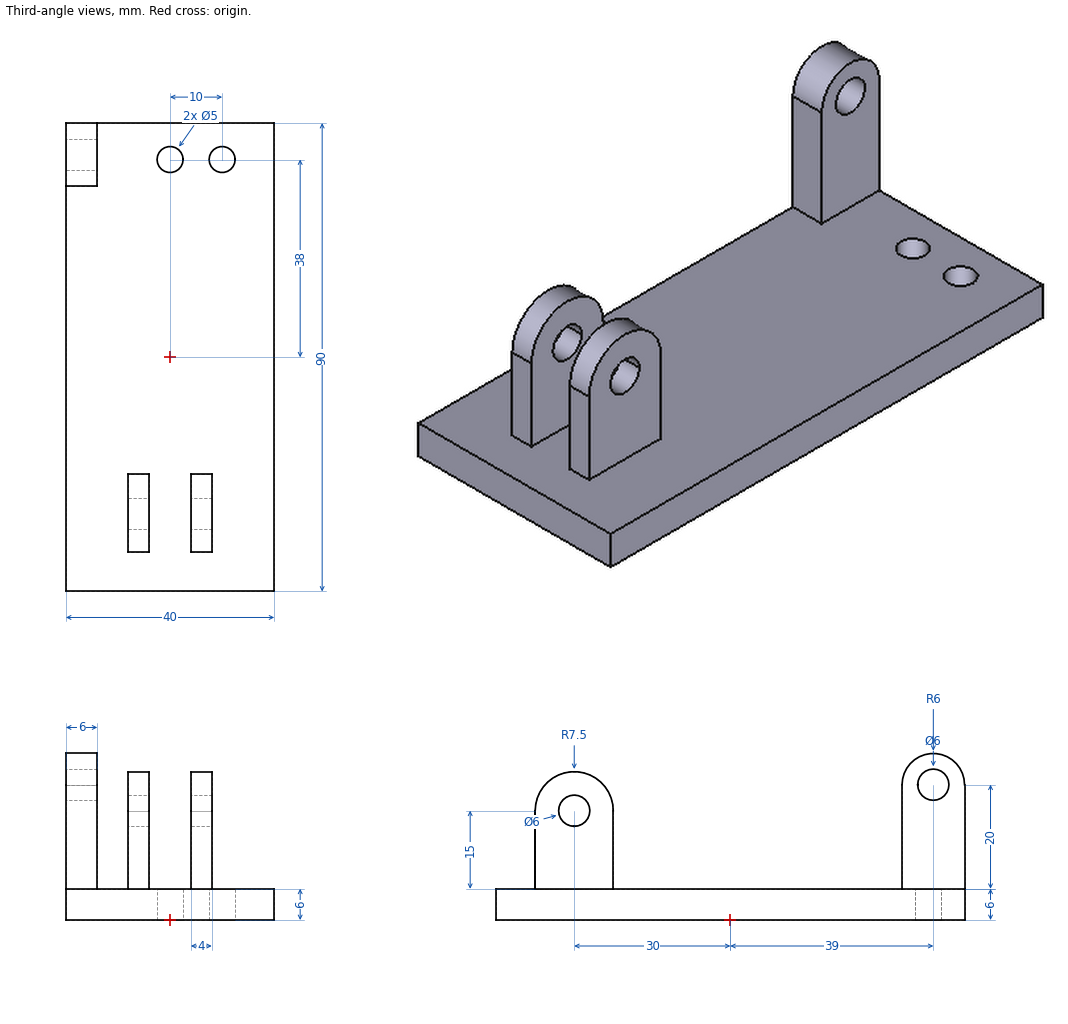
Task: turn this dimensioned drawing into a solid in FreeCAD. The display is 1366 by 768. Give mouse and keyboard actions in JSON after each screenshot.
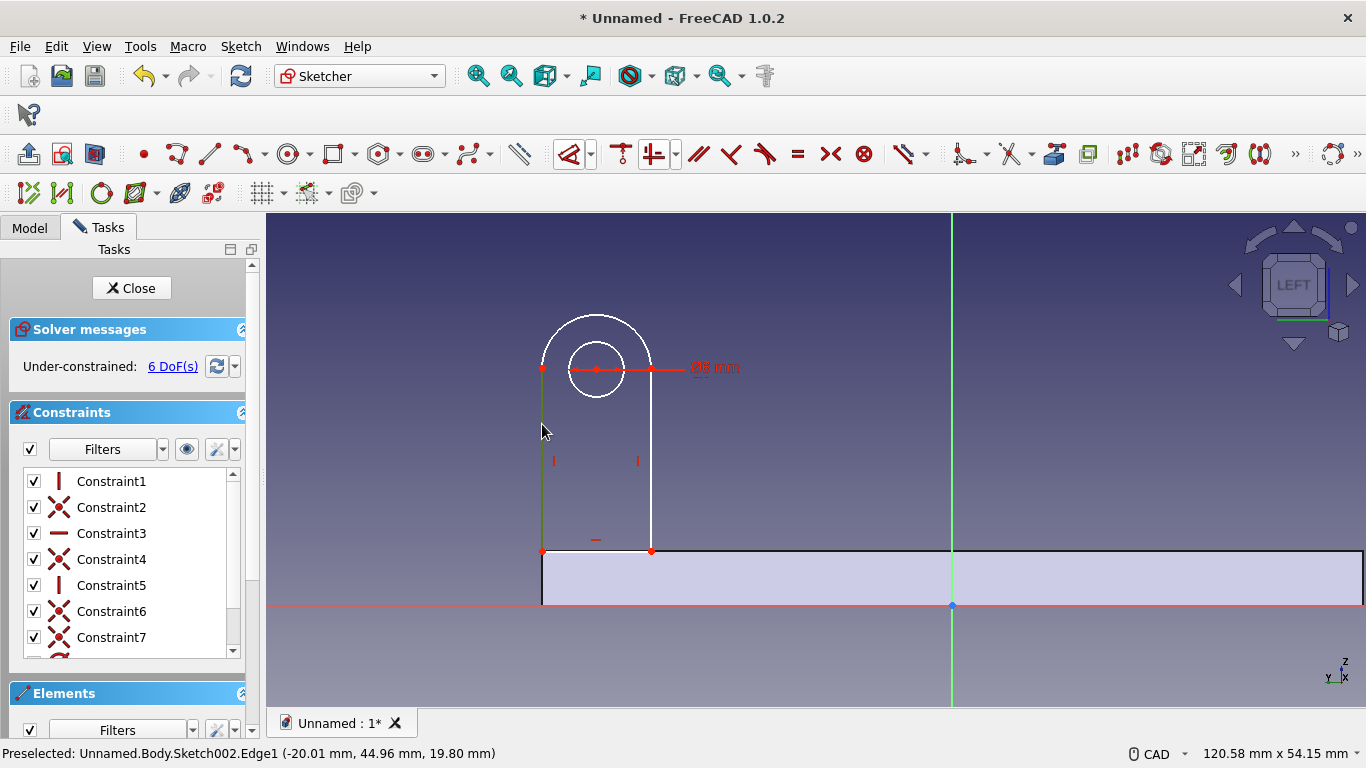
{"action": "left_click", "coordinate": [628, 325]}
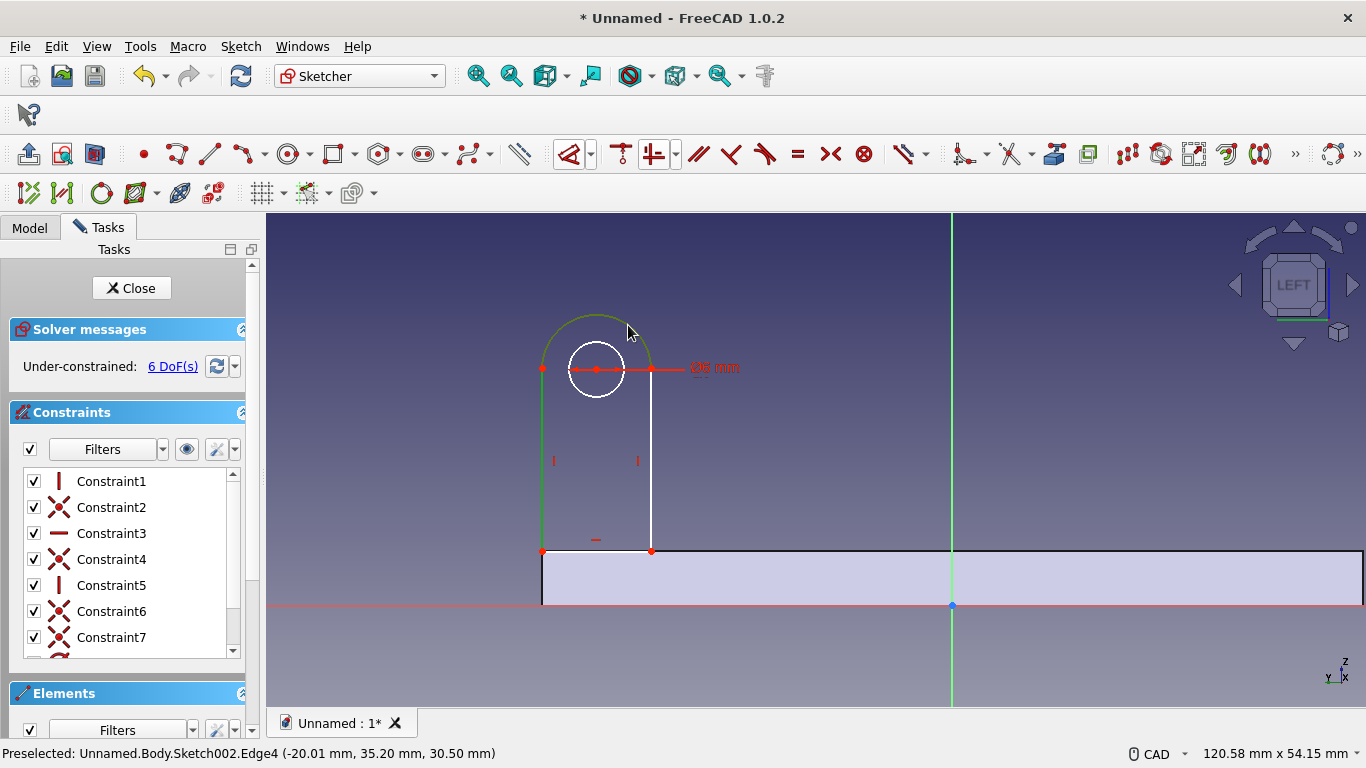
{"action": "key", "text": "t"}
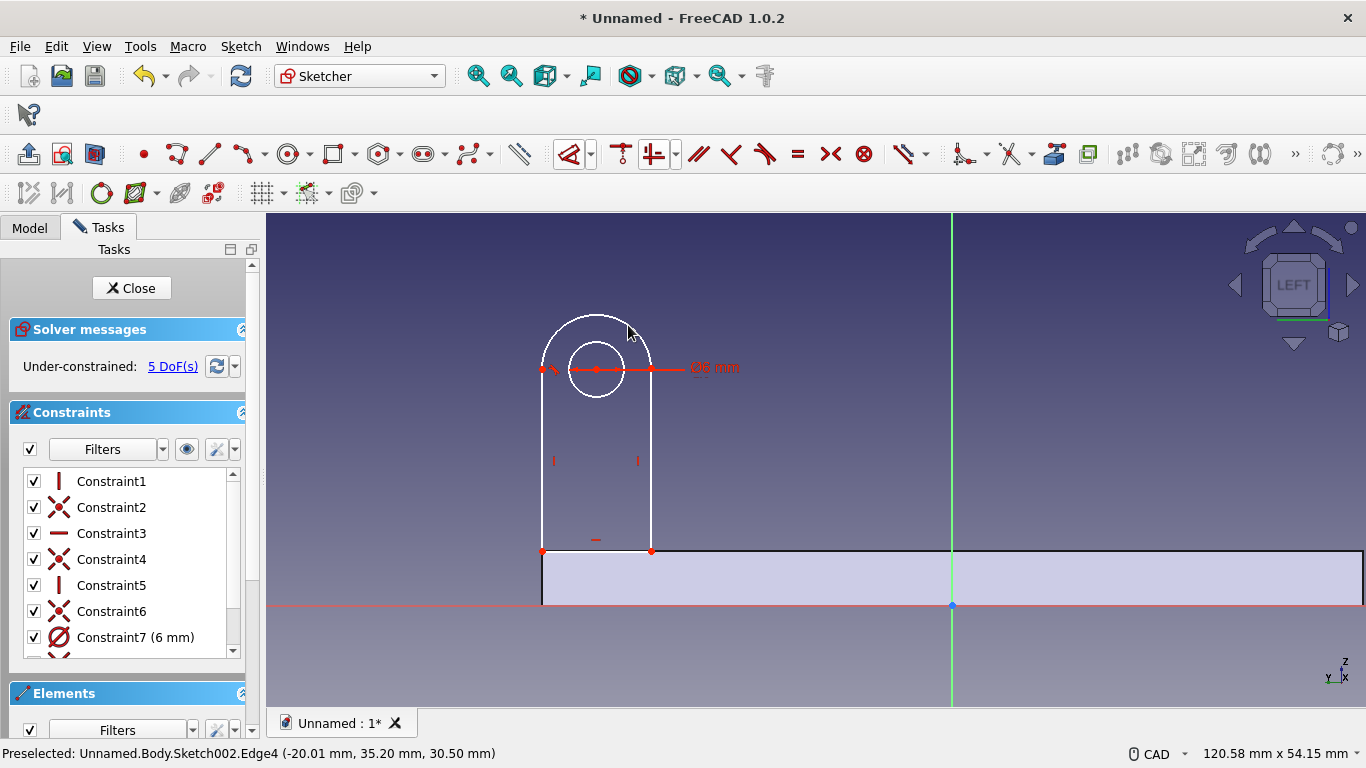
{"action": "left_click", "coordinate": [651, 497]}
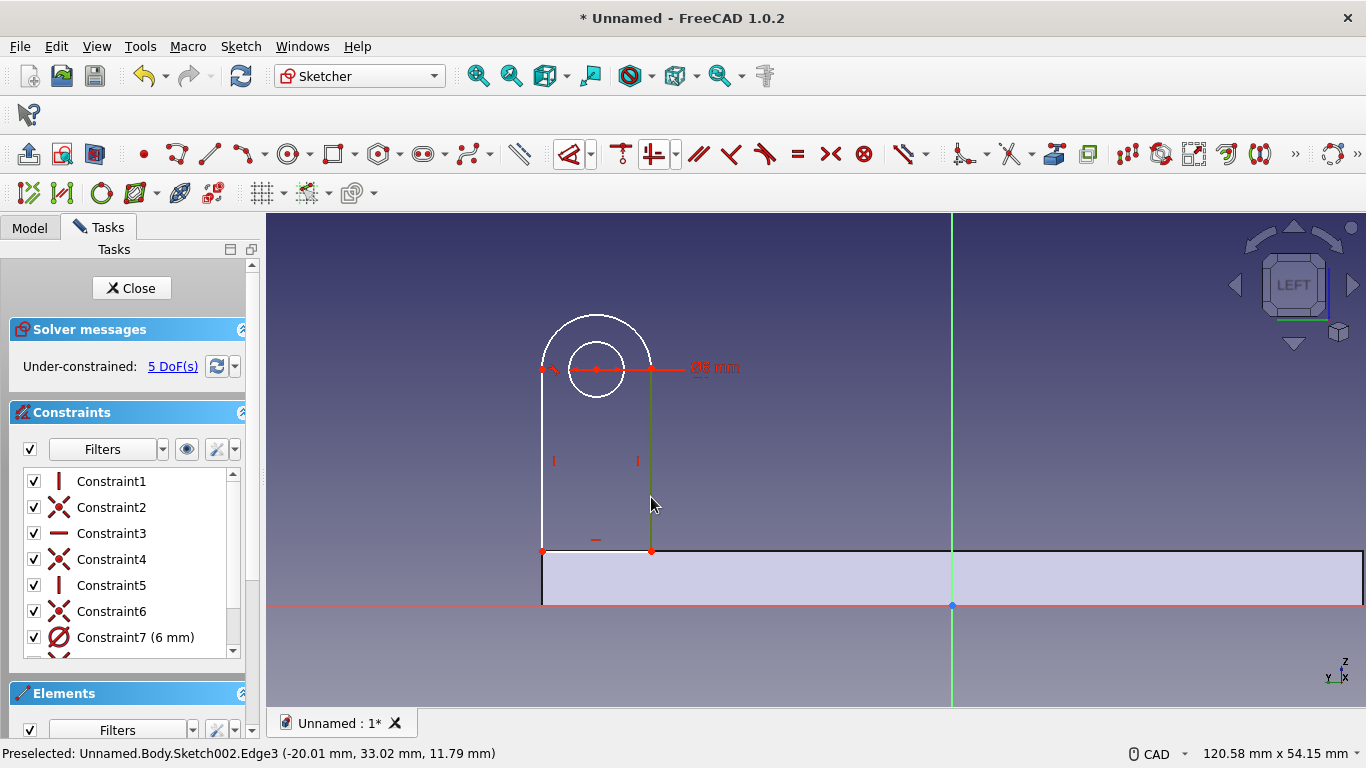
{"action": "left_click", "coordinate": [628, 325]}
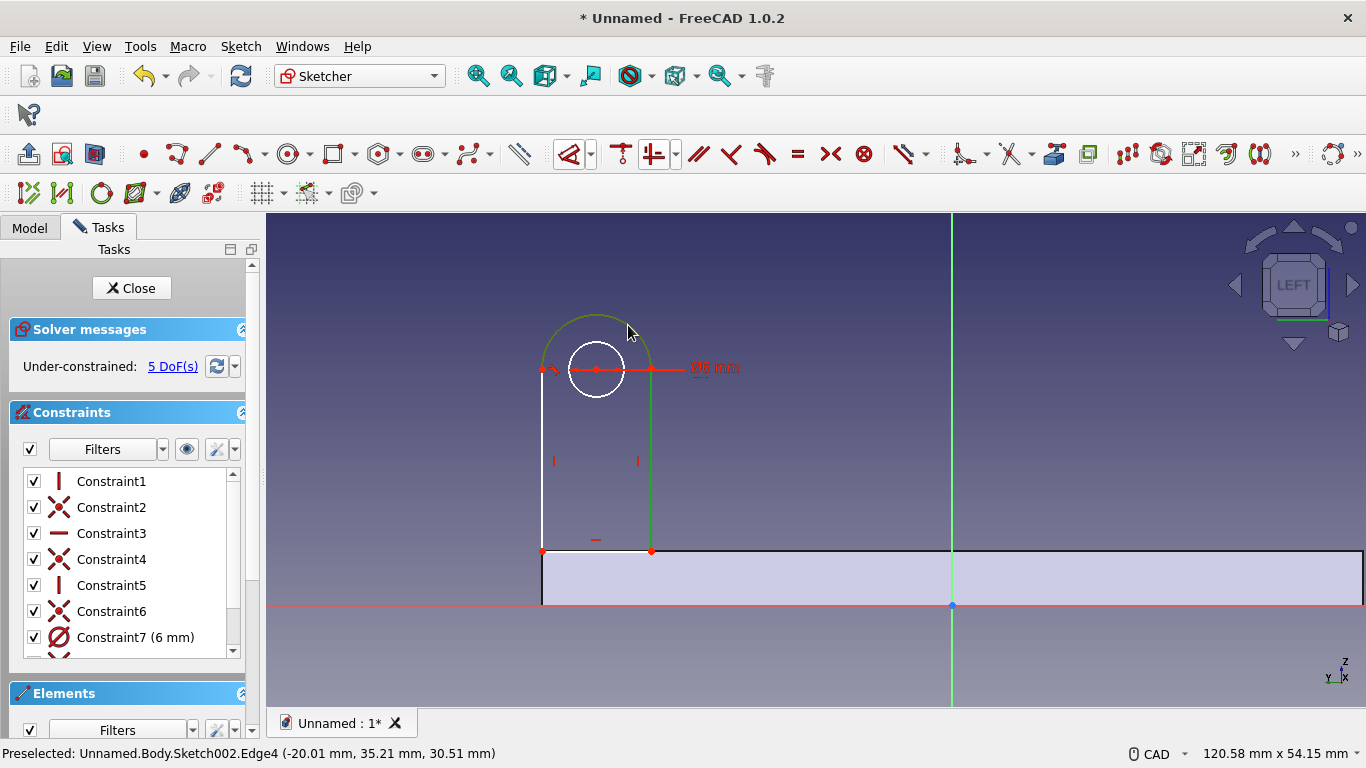
{"action": "key", "text": "t"}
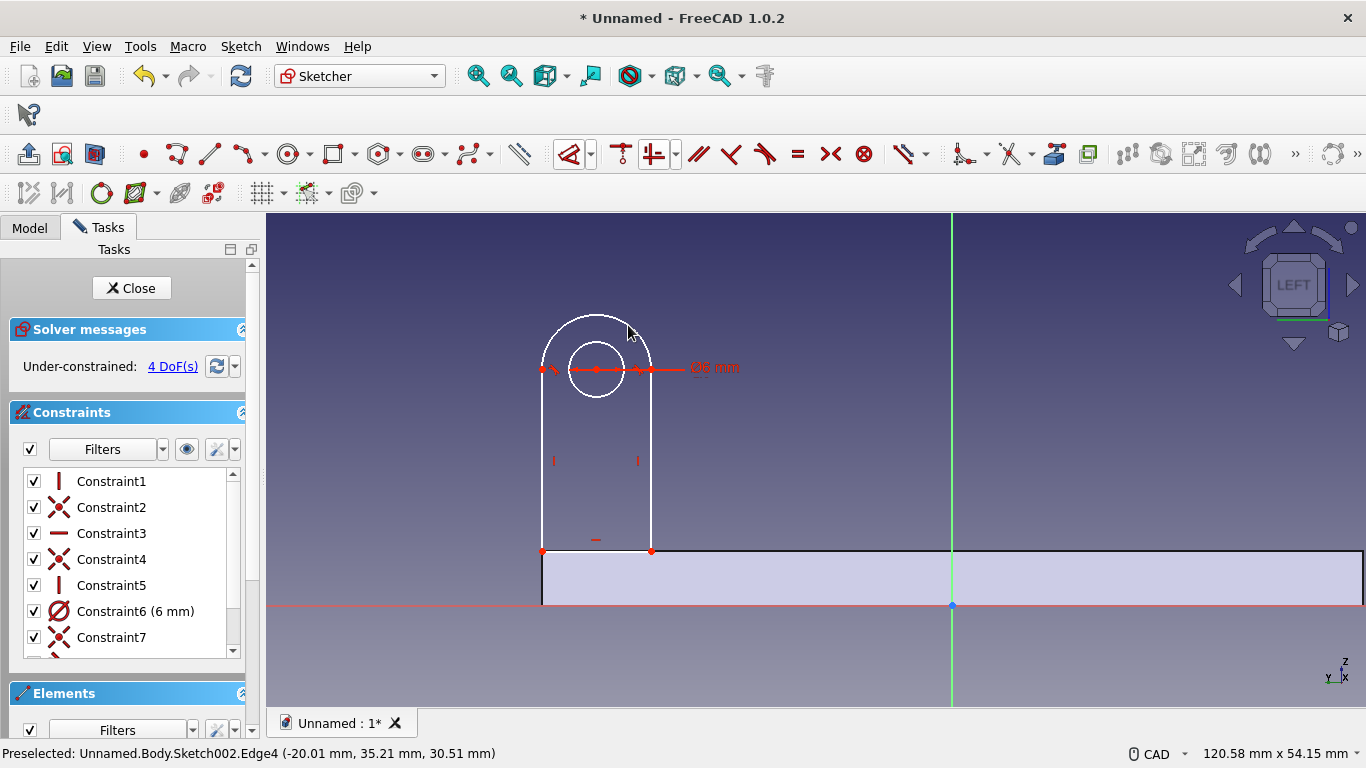
{"action": "key", "text": "d"}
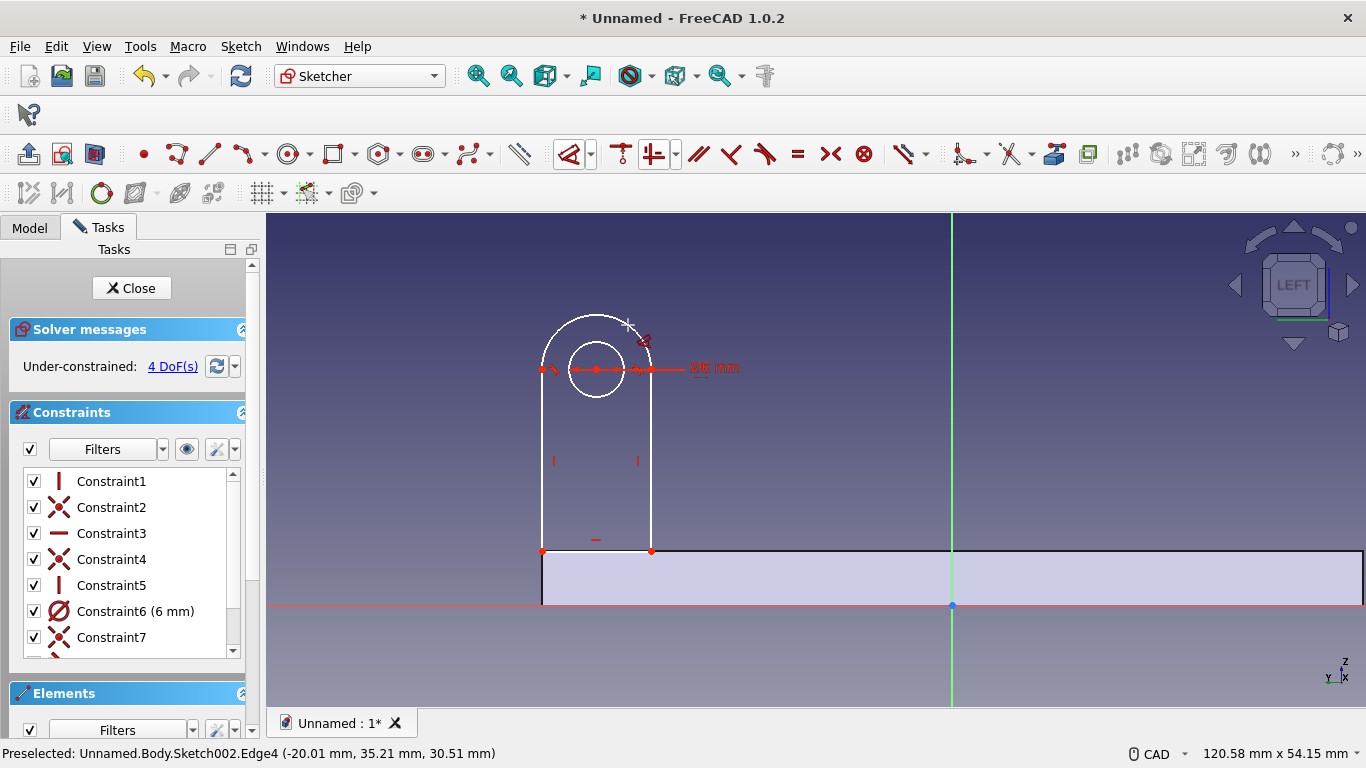
{"action": "left_click", "coordinate": [629, 325]}
{"action": "left_click", "coordinate": [648, 299]}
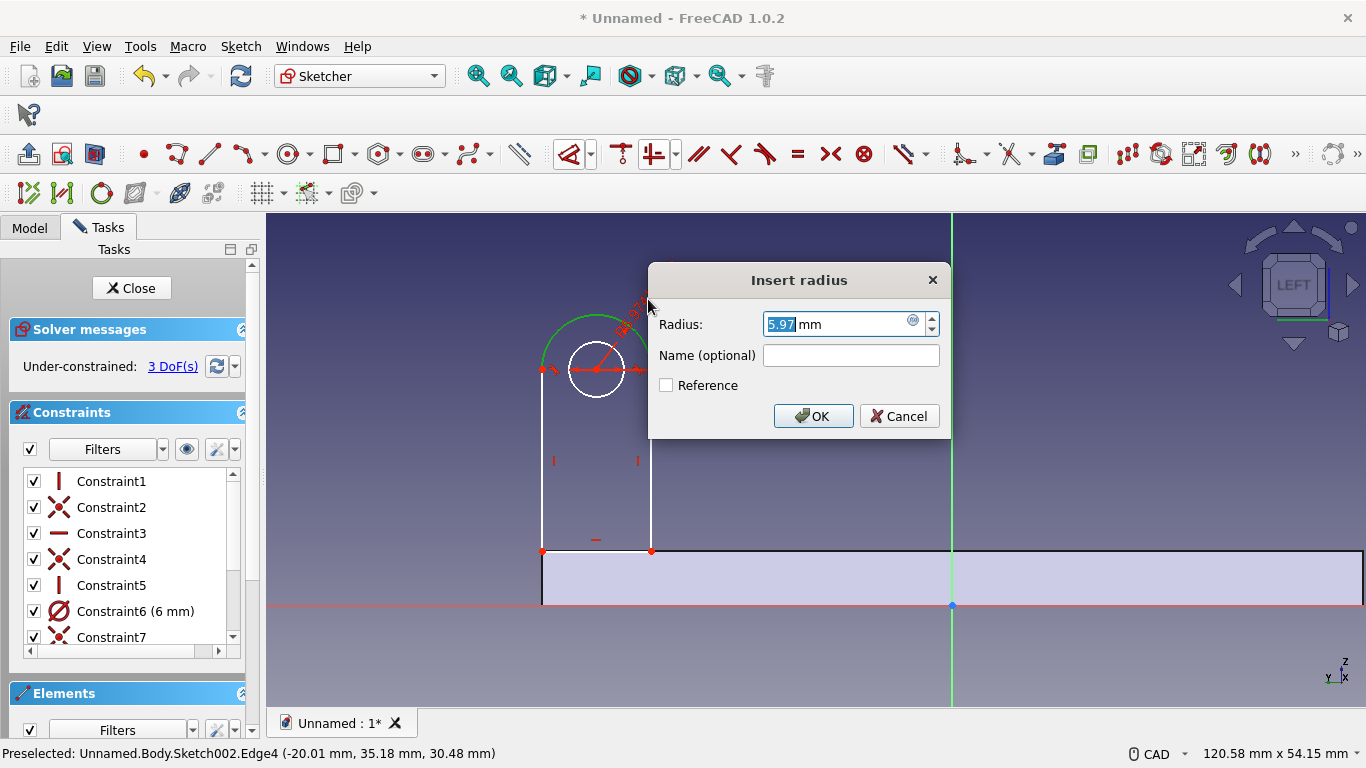
{"action": "type", "text": "6"}
{"action": "key", "text": "Return"}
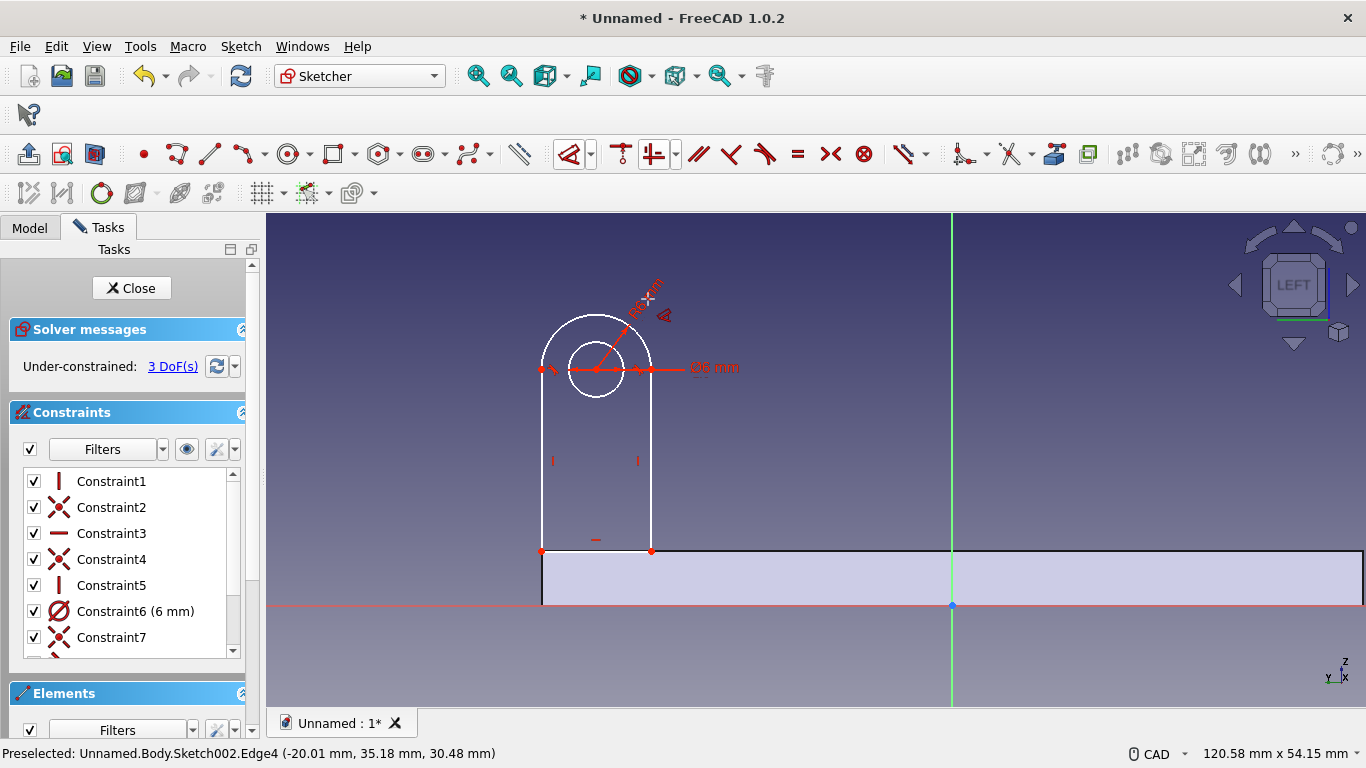
{"action": "left_click", "coordinate": [542, 424]}
{"action": "left_click", "coordinate": [508, 461]}